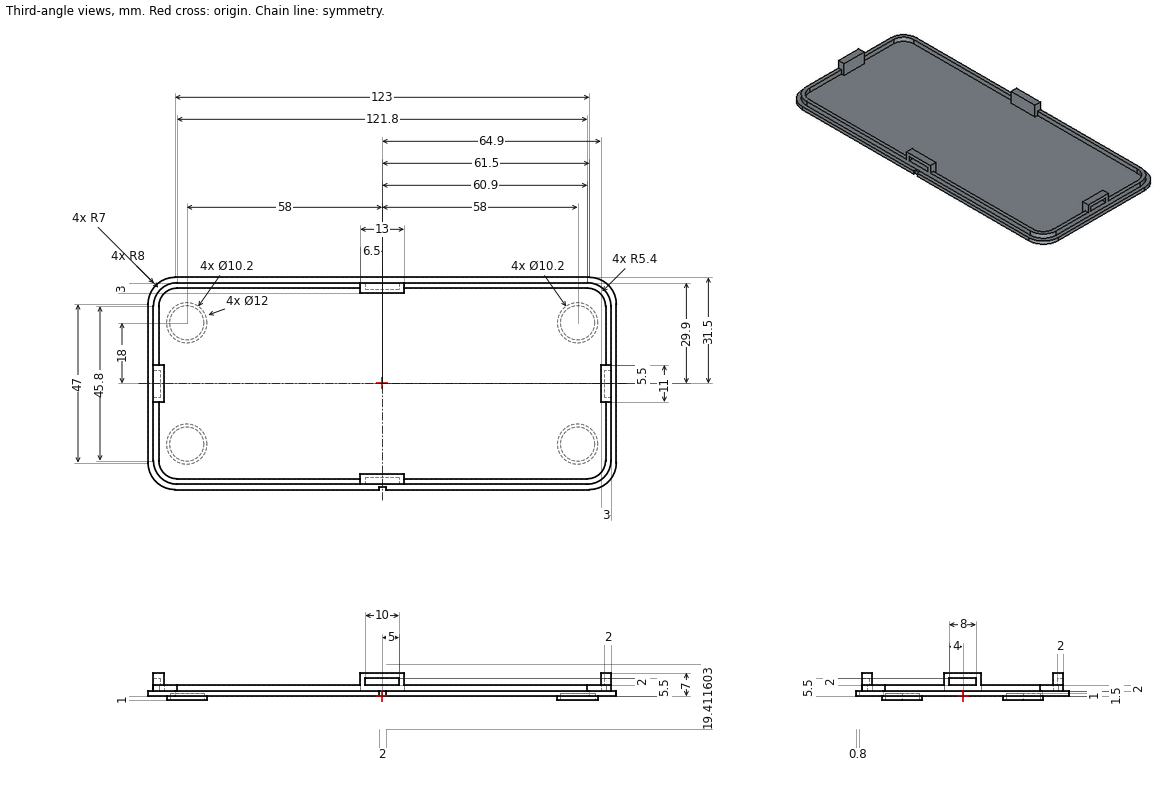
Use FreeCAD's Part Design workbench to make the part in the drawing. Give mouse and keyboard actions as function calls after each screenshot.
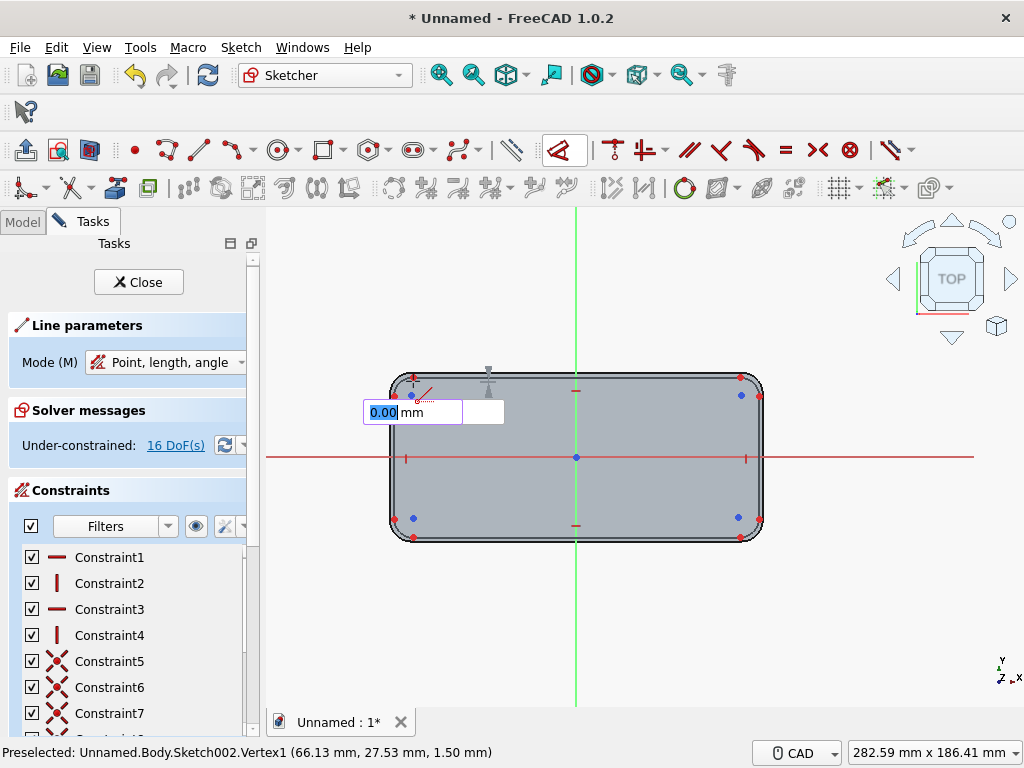
scroll(740, 381, up, 7)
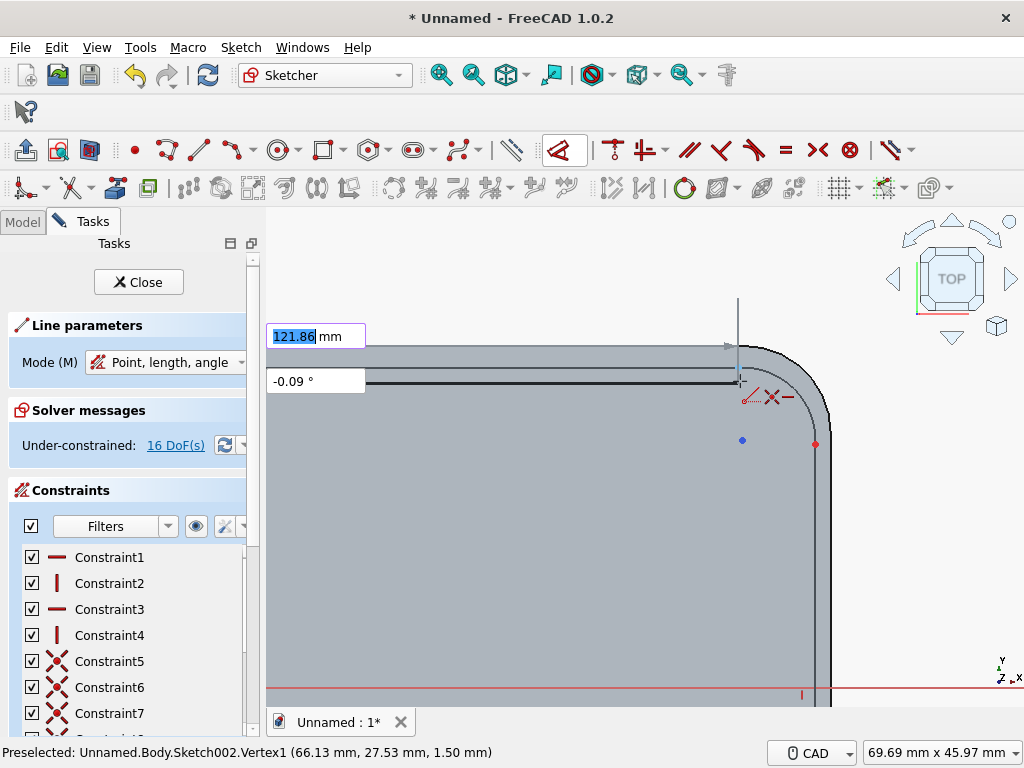
click(737, 381)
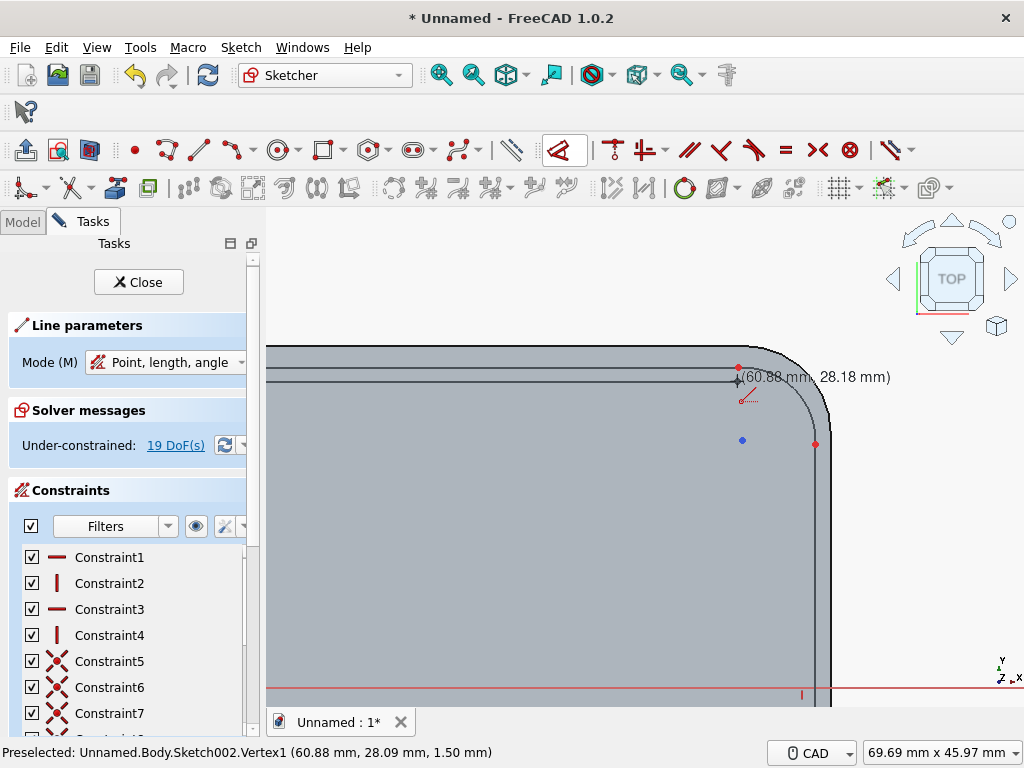
click(796, 439)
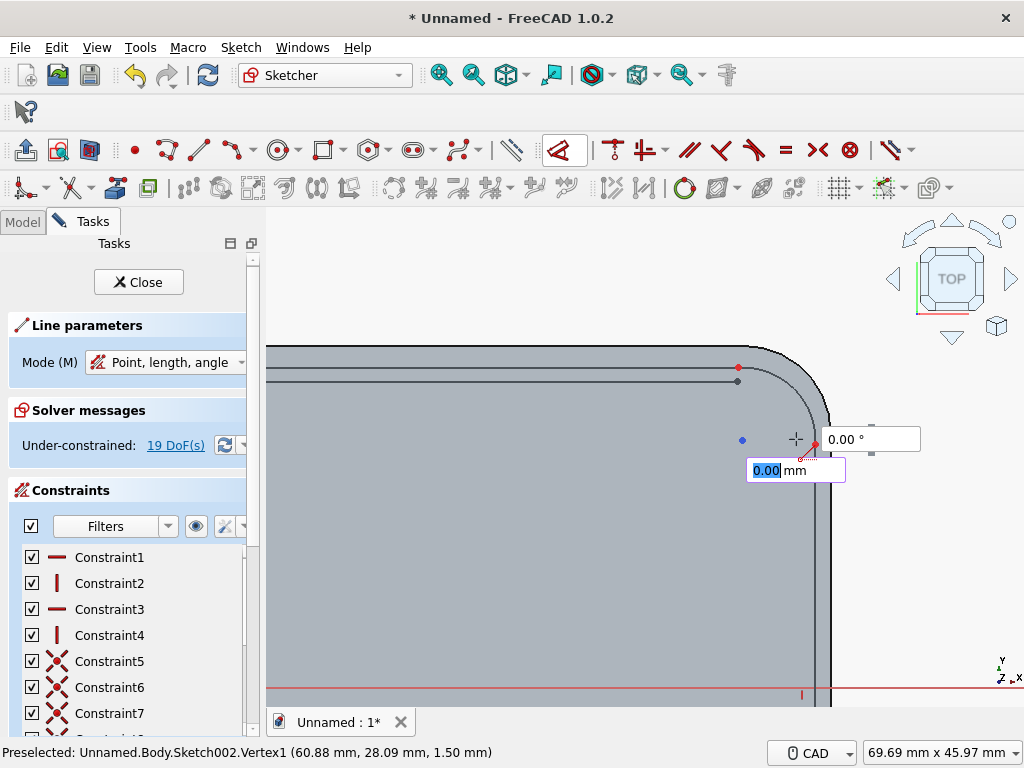
scroll(741, 381, down, 7)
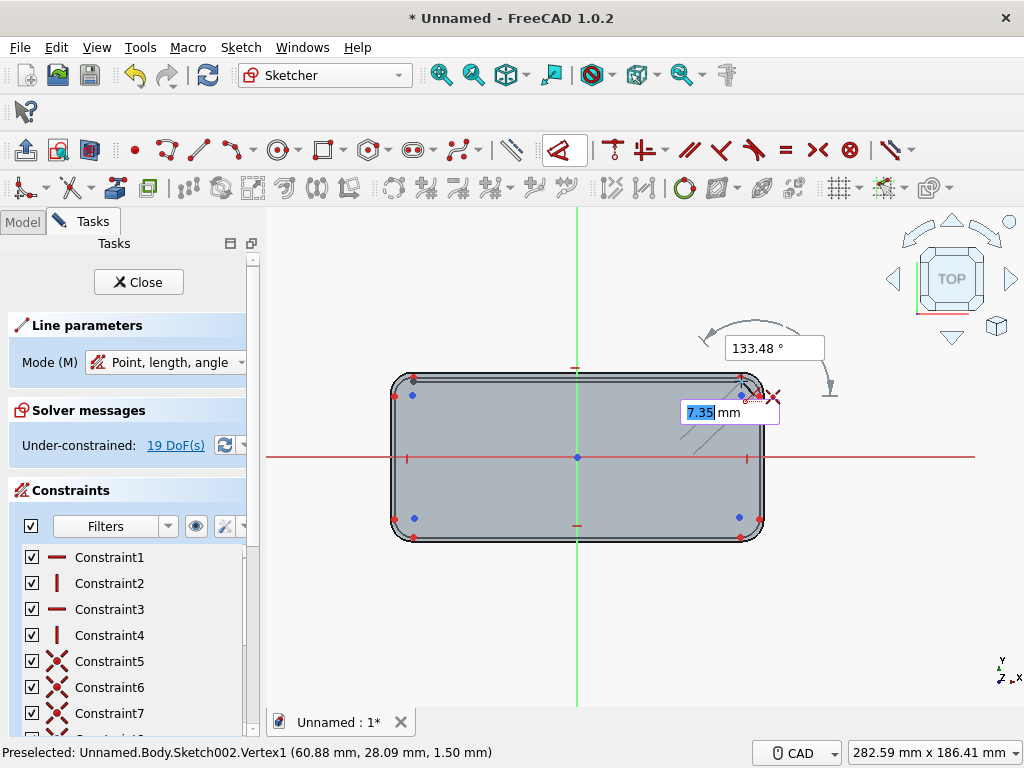
scroll(755, 519, up, 7)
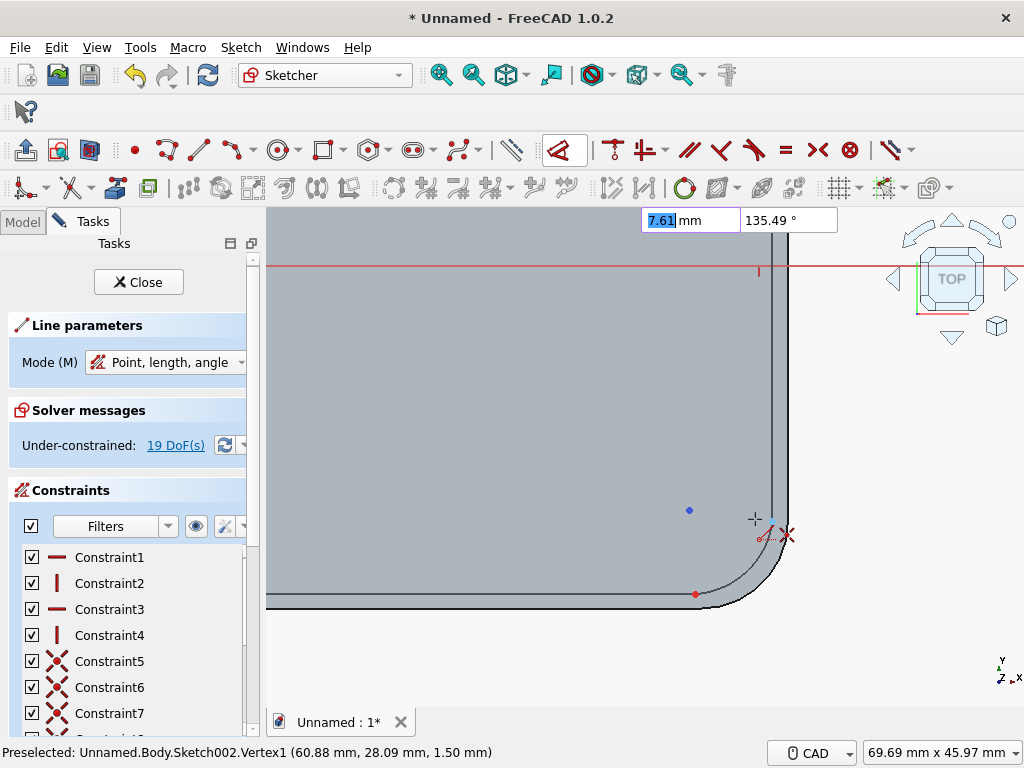
click(753, 515)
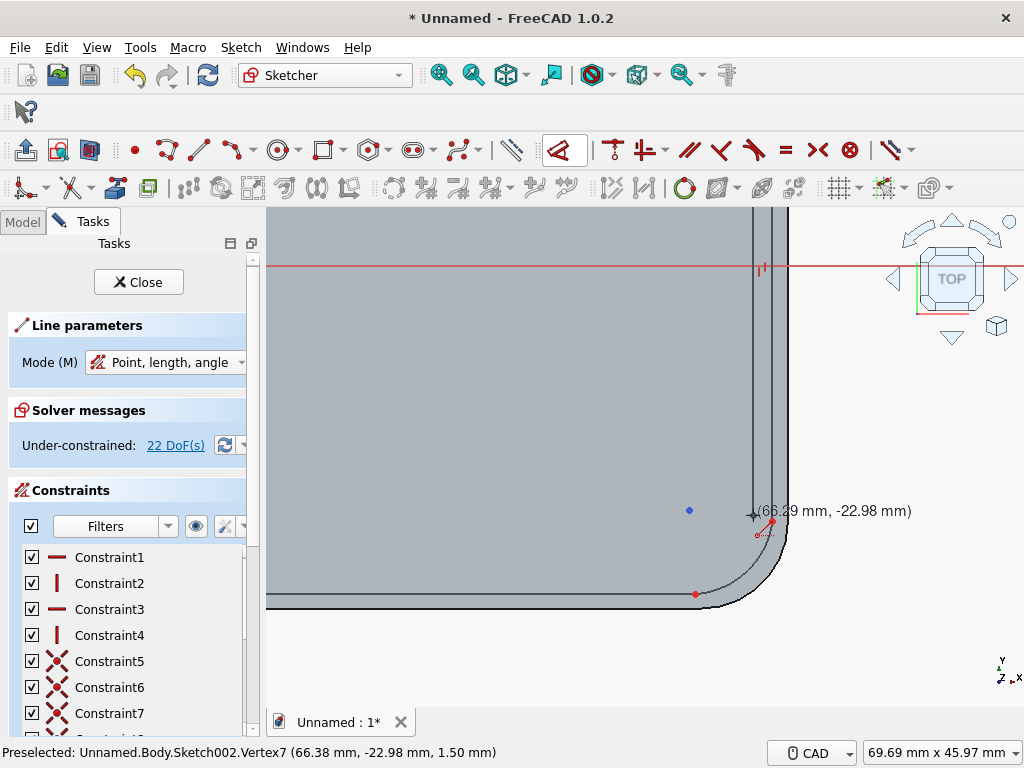
click(694, 574)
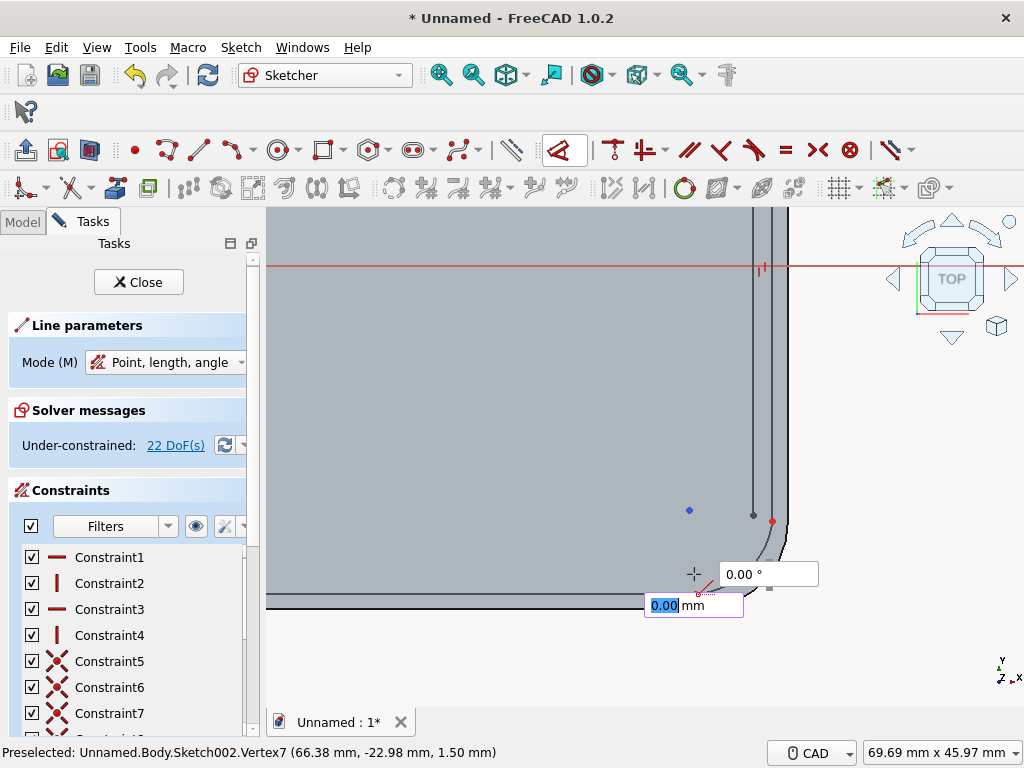
scroll(755, 520, down, 7)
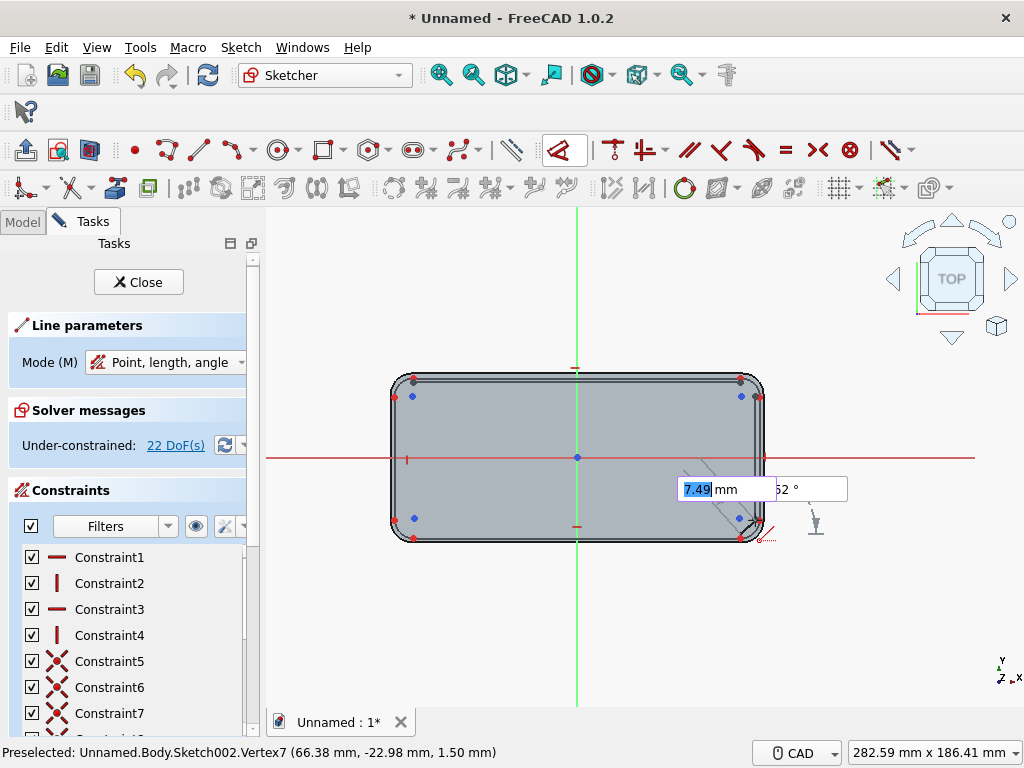
scroll(414, 534, up, 7)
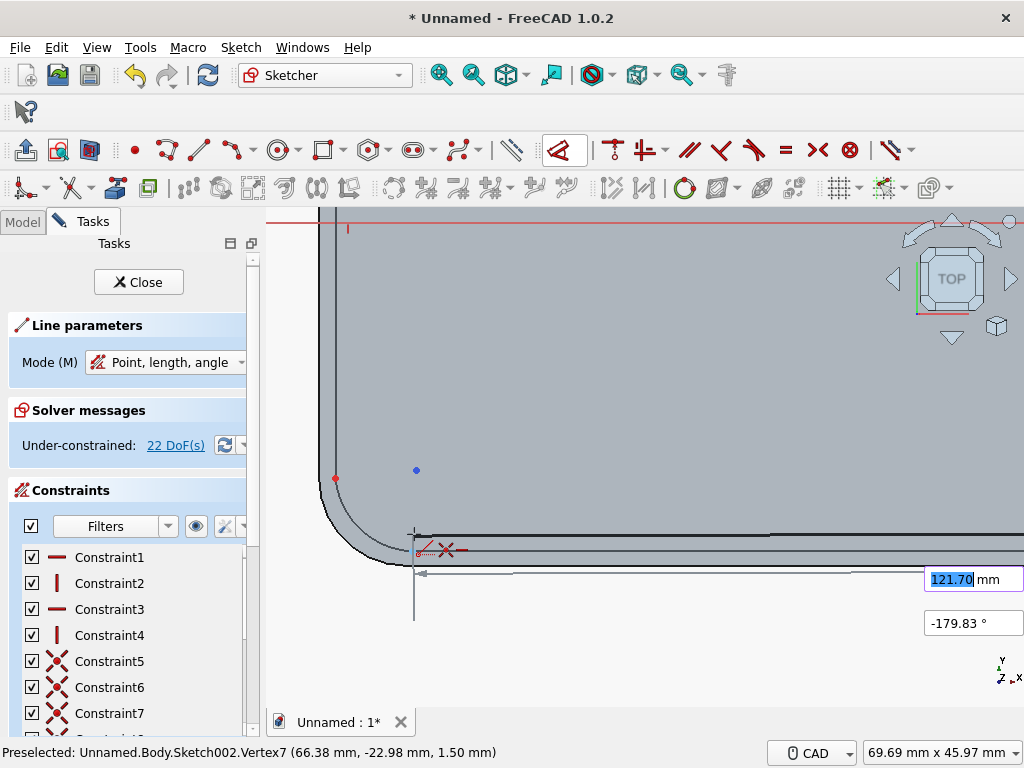
click(413, 531)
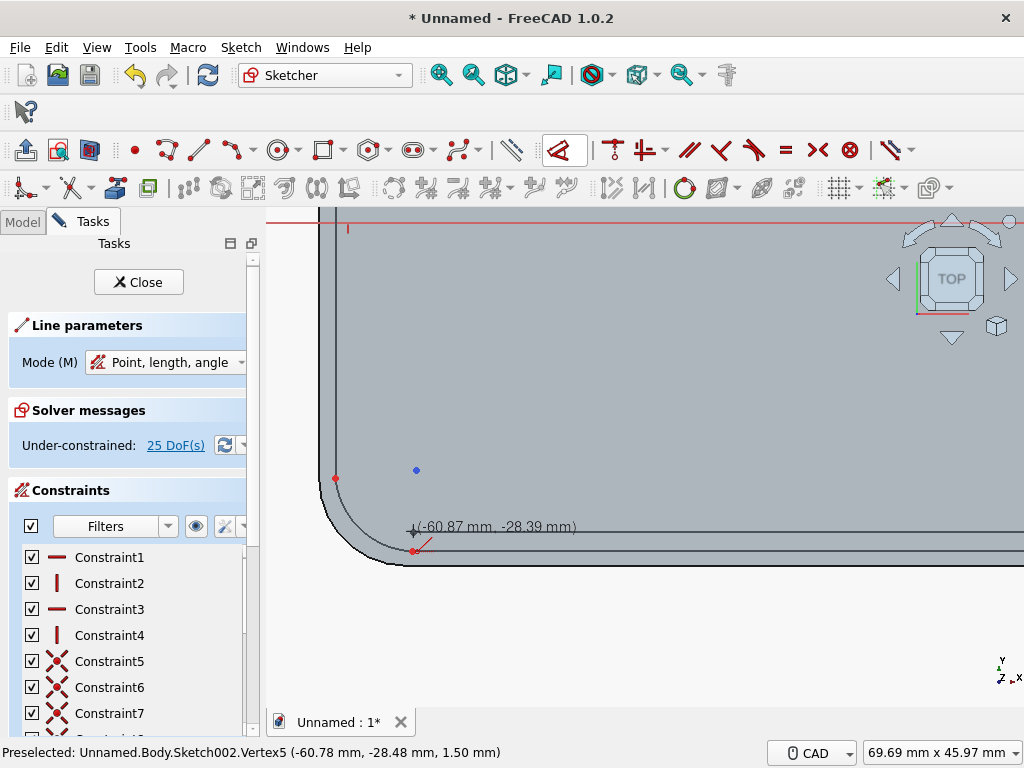
click(354, 472)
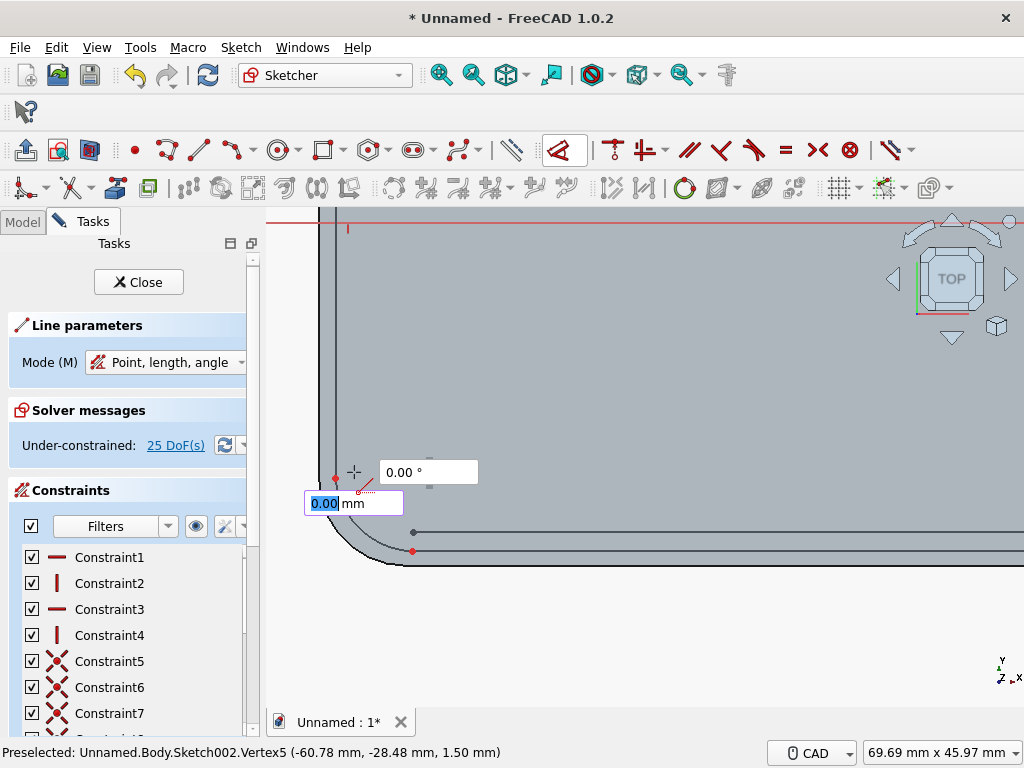
scroll(413, 534, down, 7)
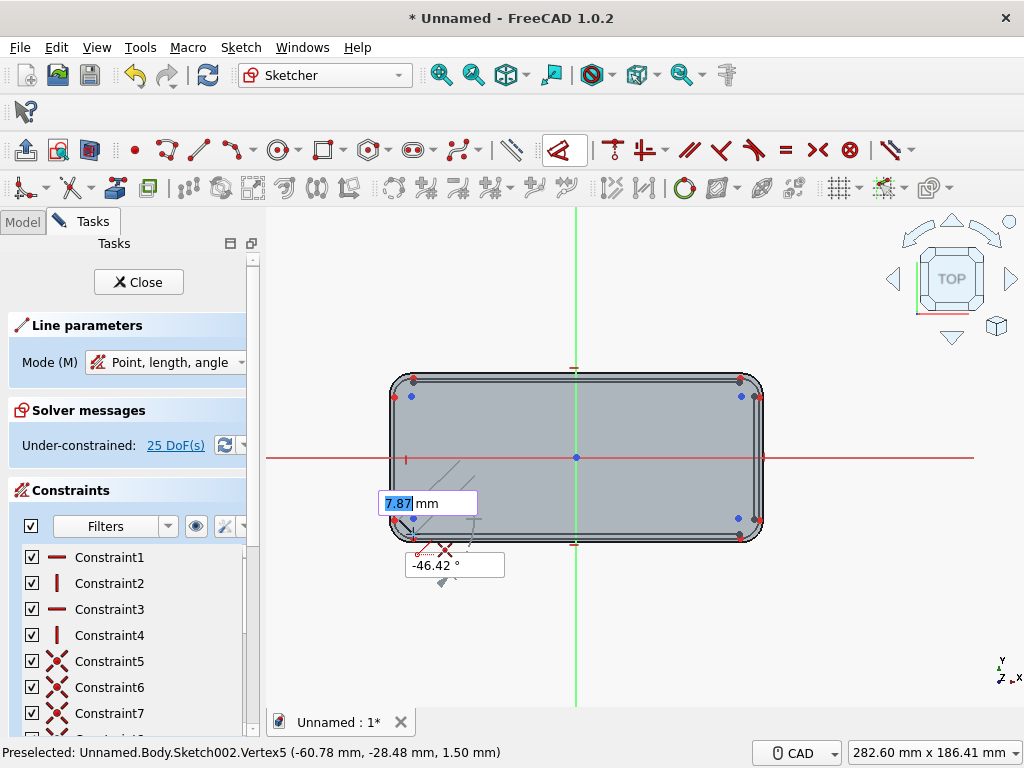
scroll(399, 396, up, 7)